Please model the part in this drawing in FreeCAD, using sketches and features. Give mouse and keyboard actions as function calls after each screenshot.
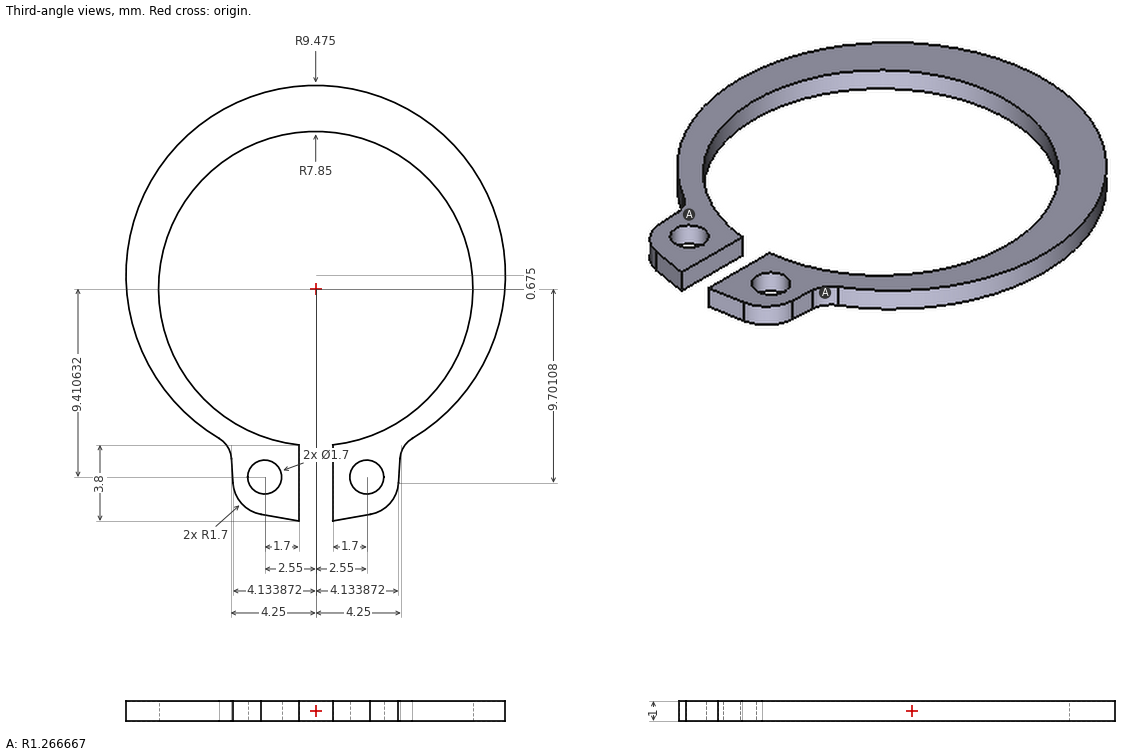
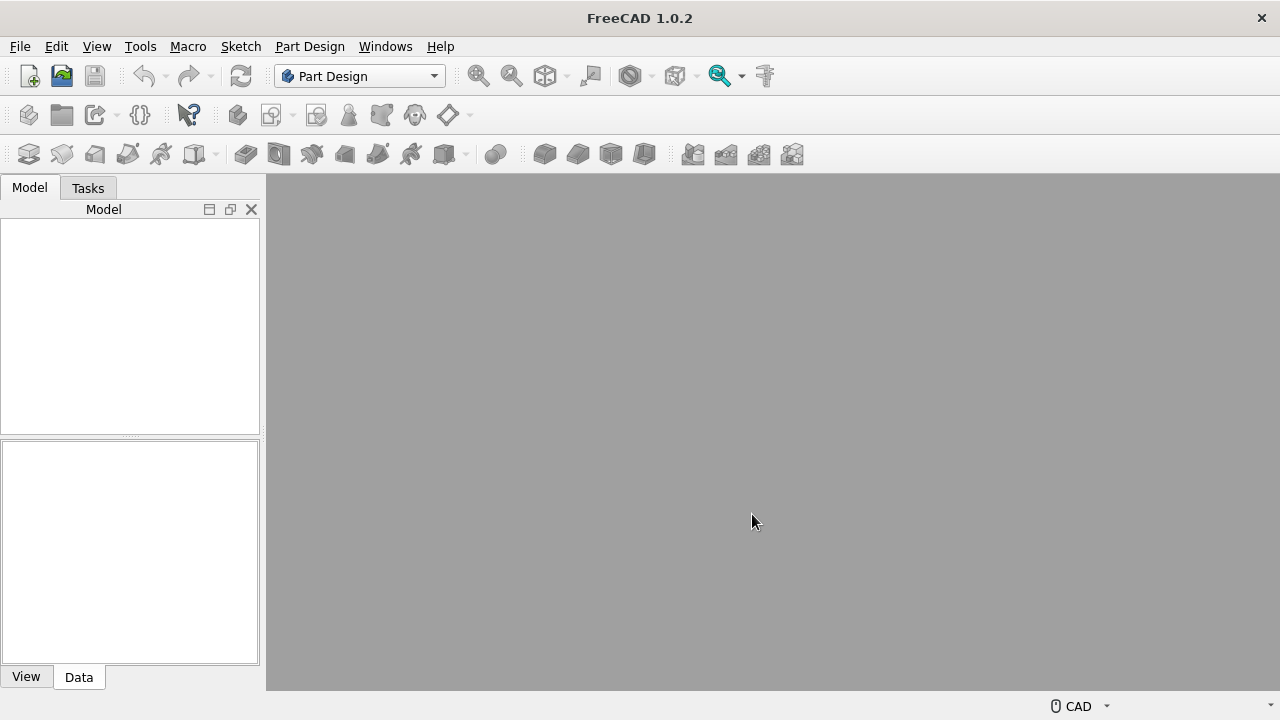
click(29, 76)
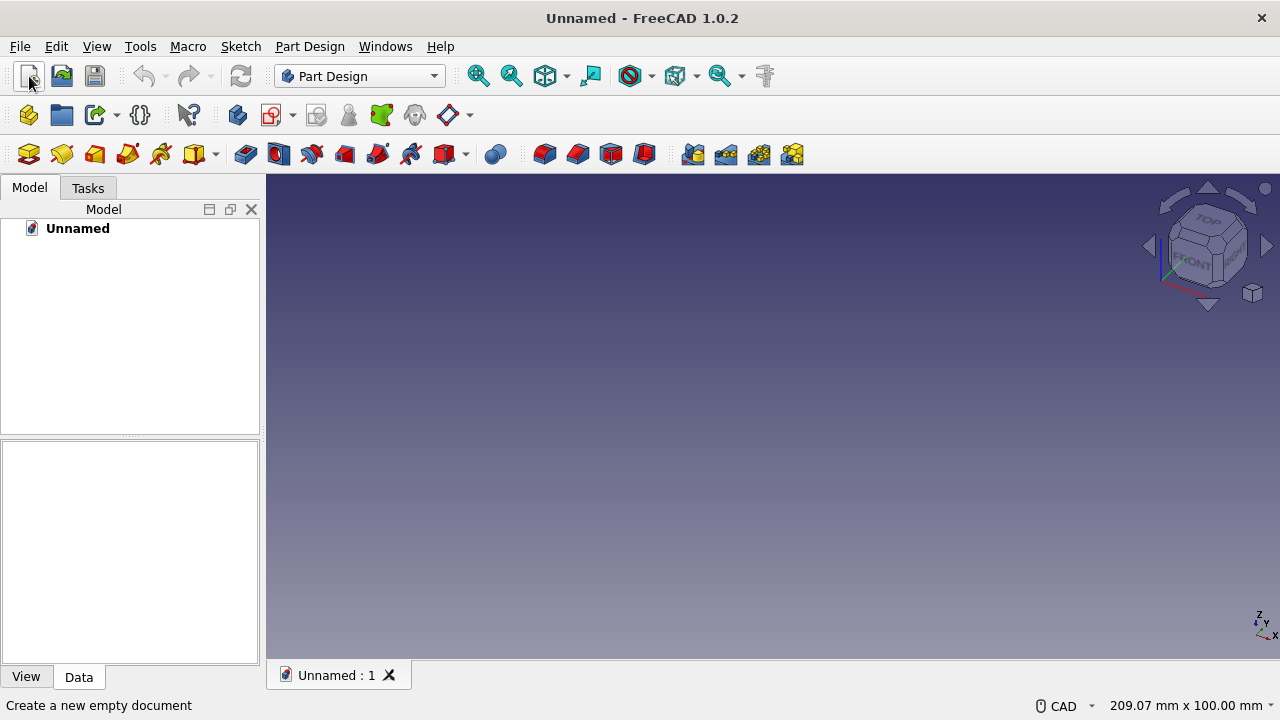
click(270, 116)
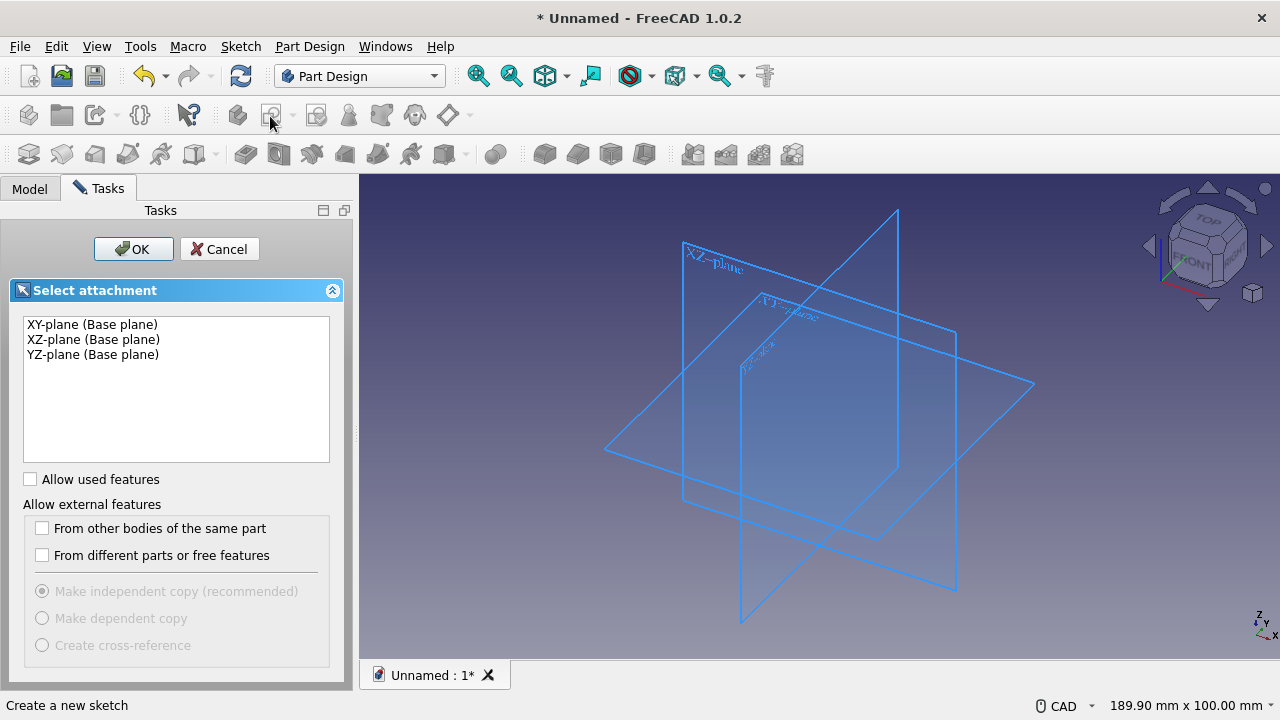
click(84, 324)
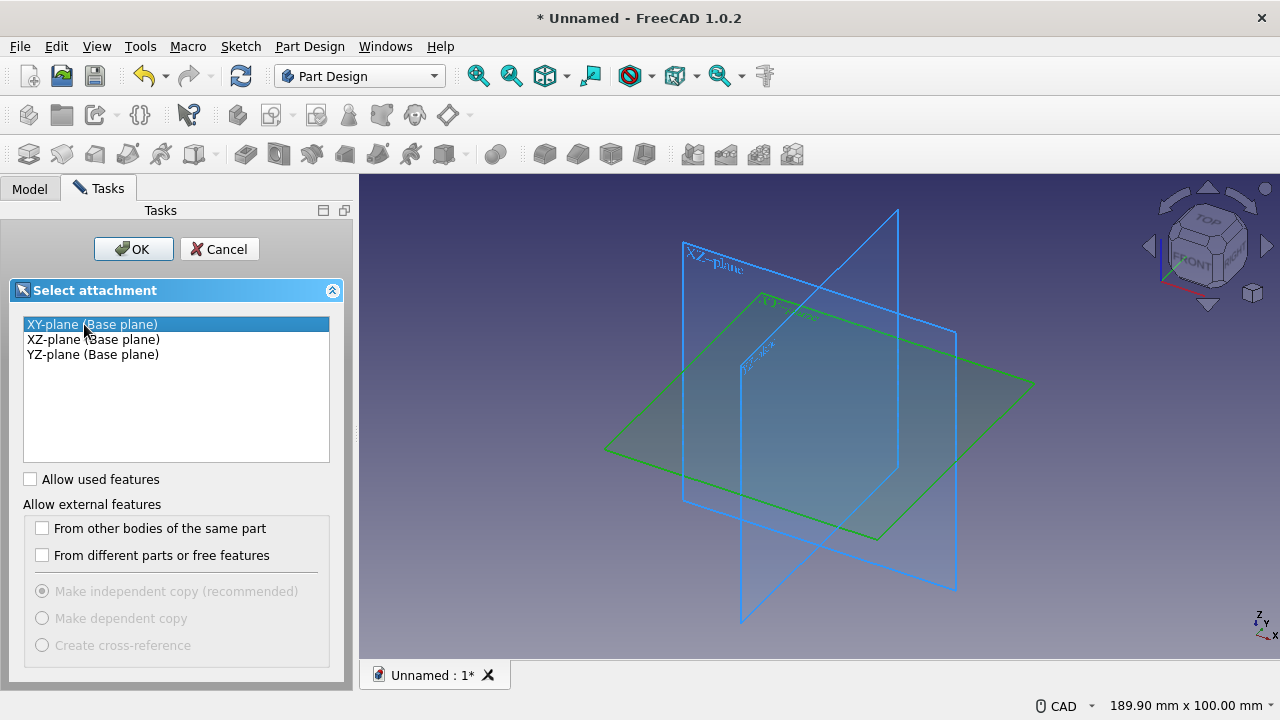
click(134, 249)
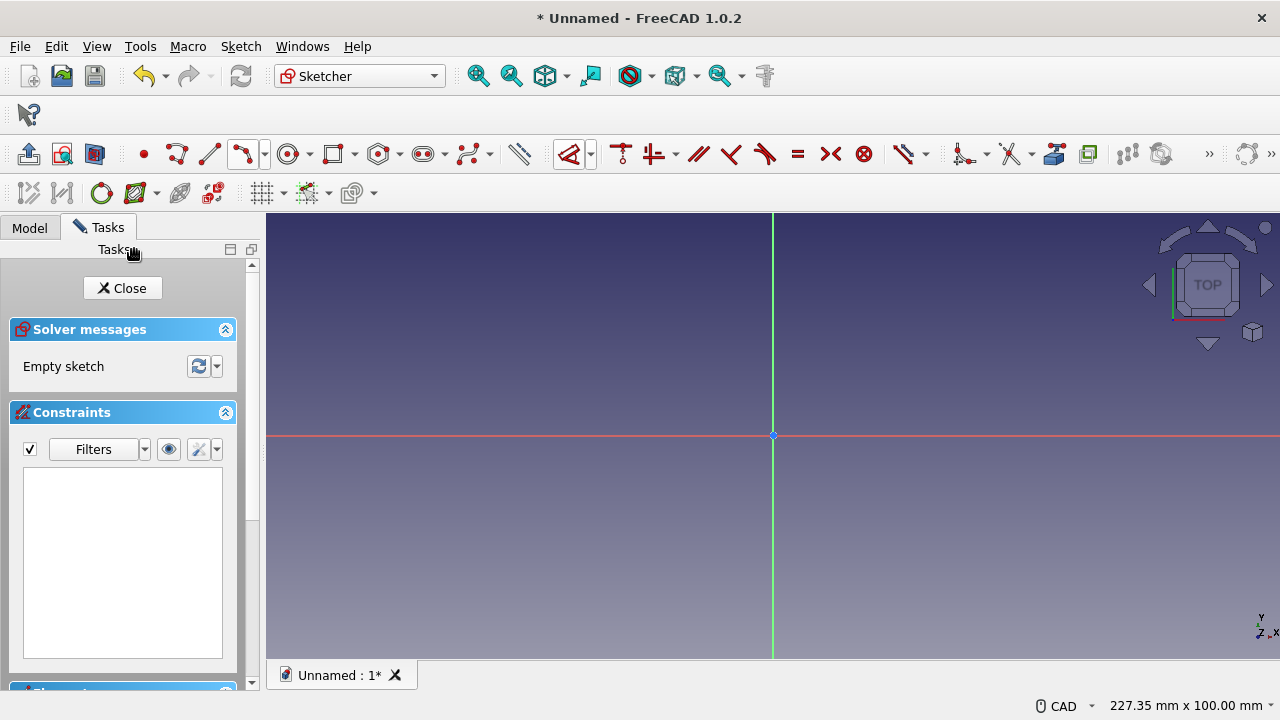
scroll(813, 441, up, 5)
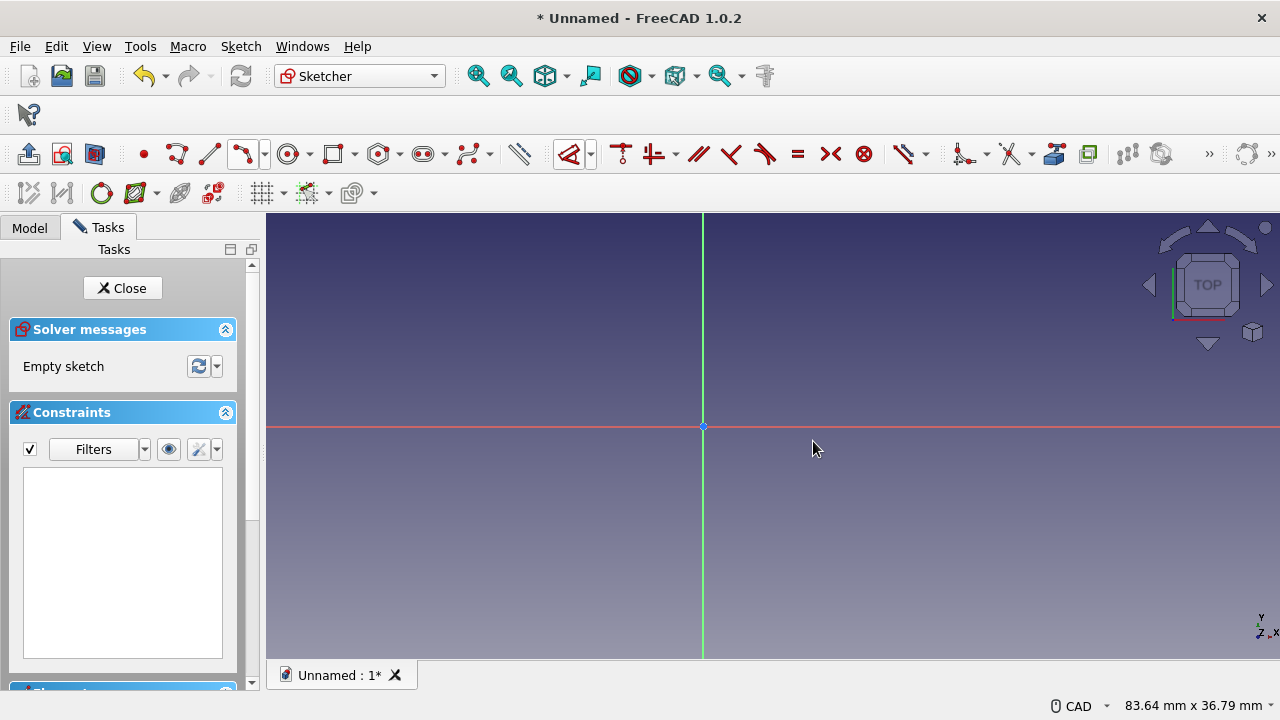
click(210, 154)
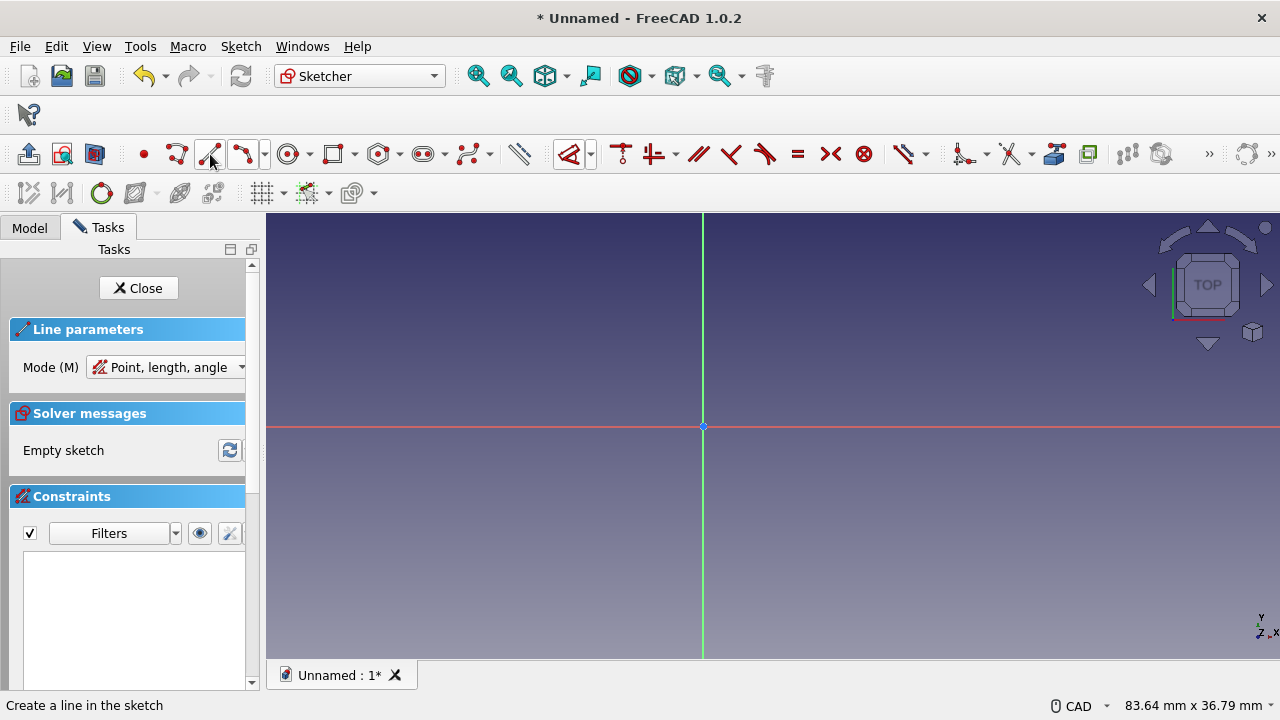
click(753, 544)
click(756, 521)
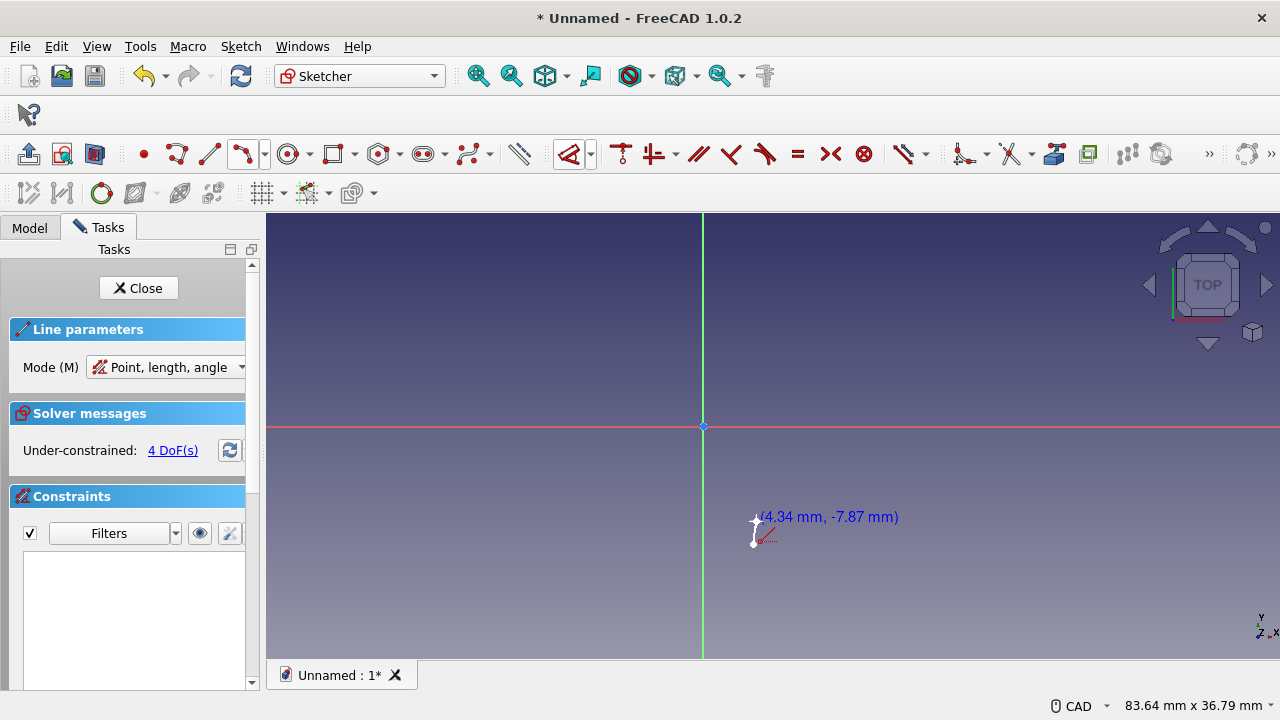
click(652, 521)
click(655, 544)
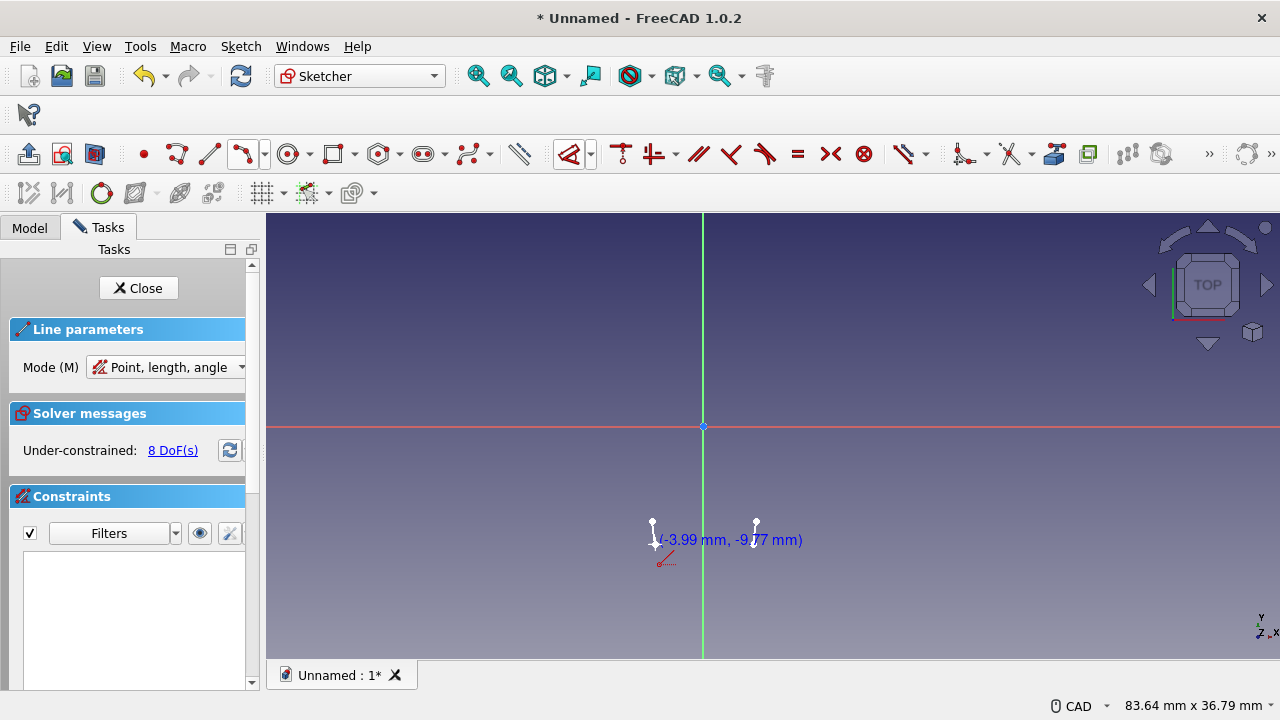
click(177, 154)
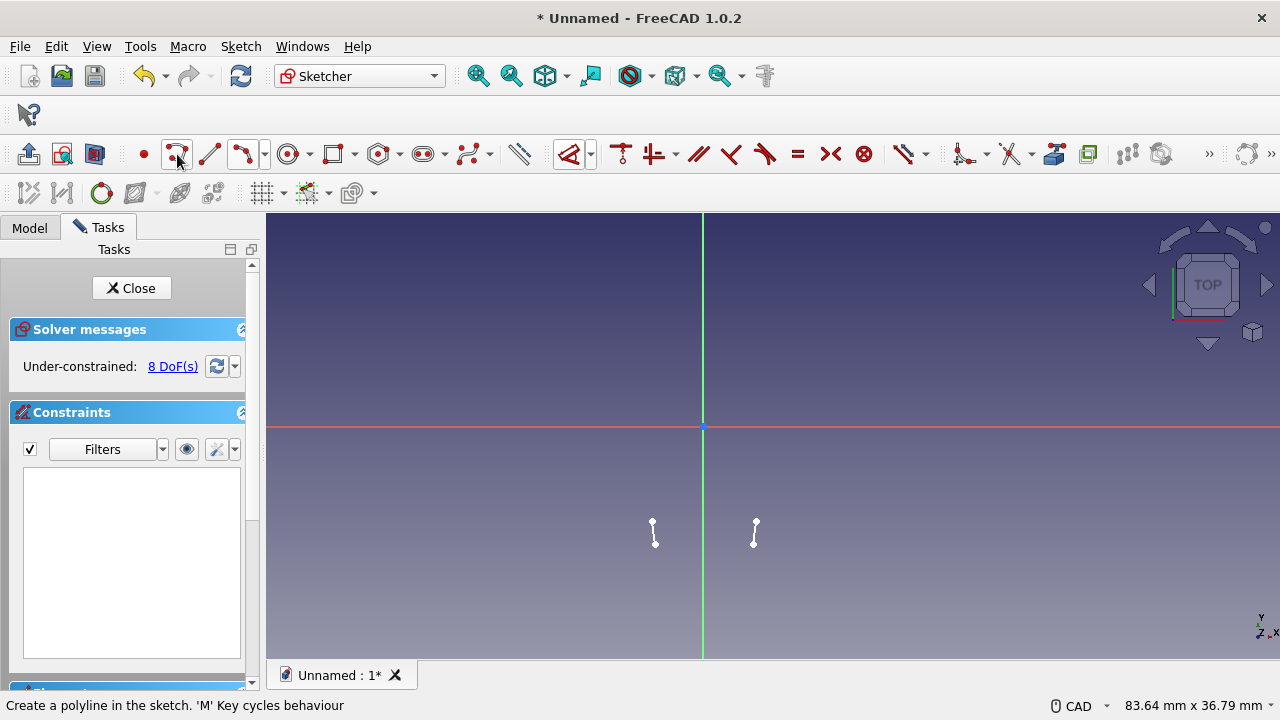
click(670, 563)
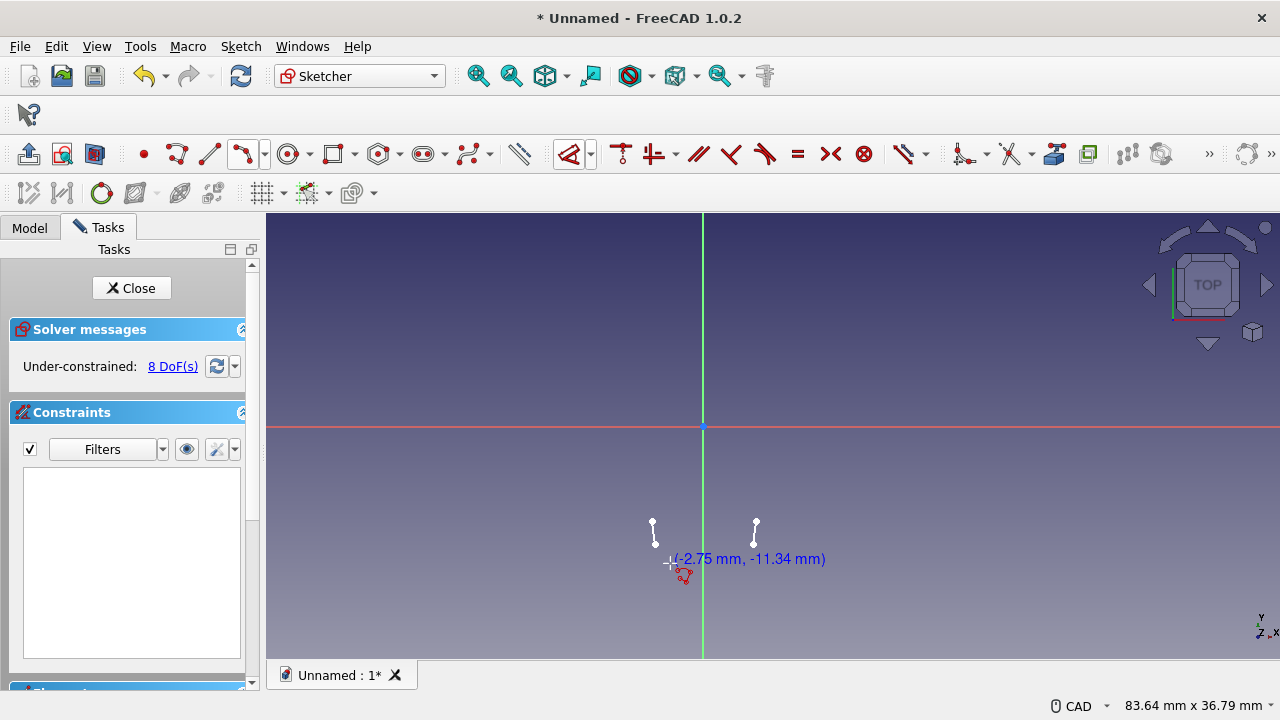
scroll(693, 567, up, 3)